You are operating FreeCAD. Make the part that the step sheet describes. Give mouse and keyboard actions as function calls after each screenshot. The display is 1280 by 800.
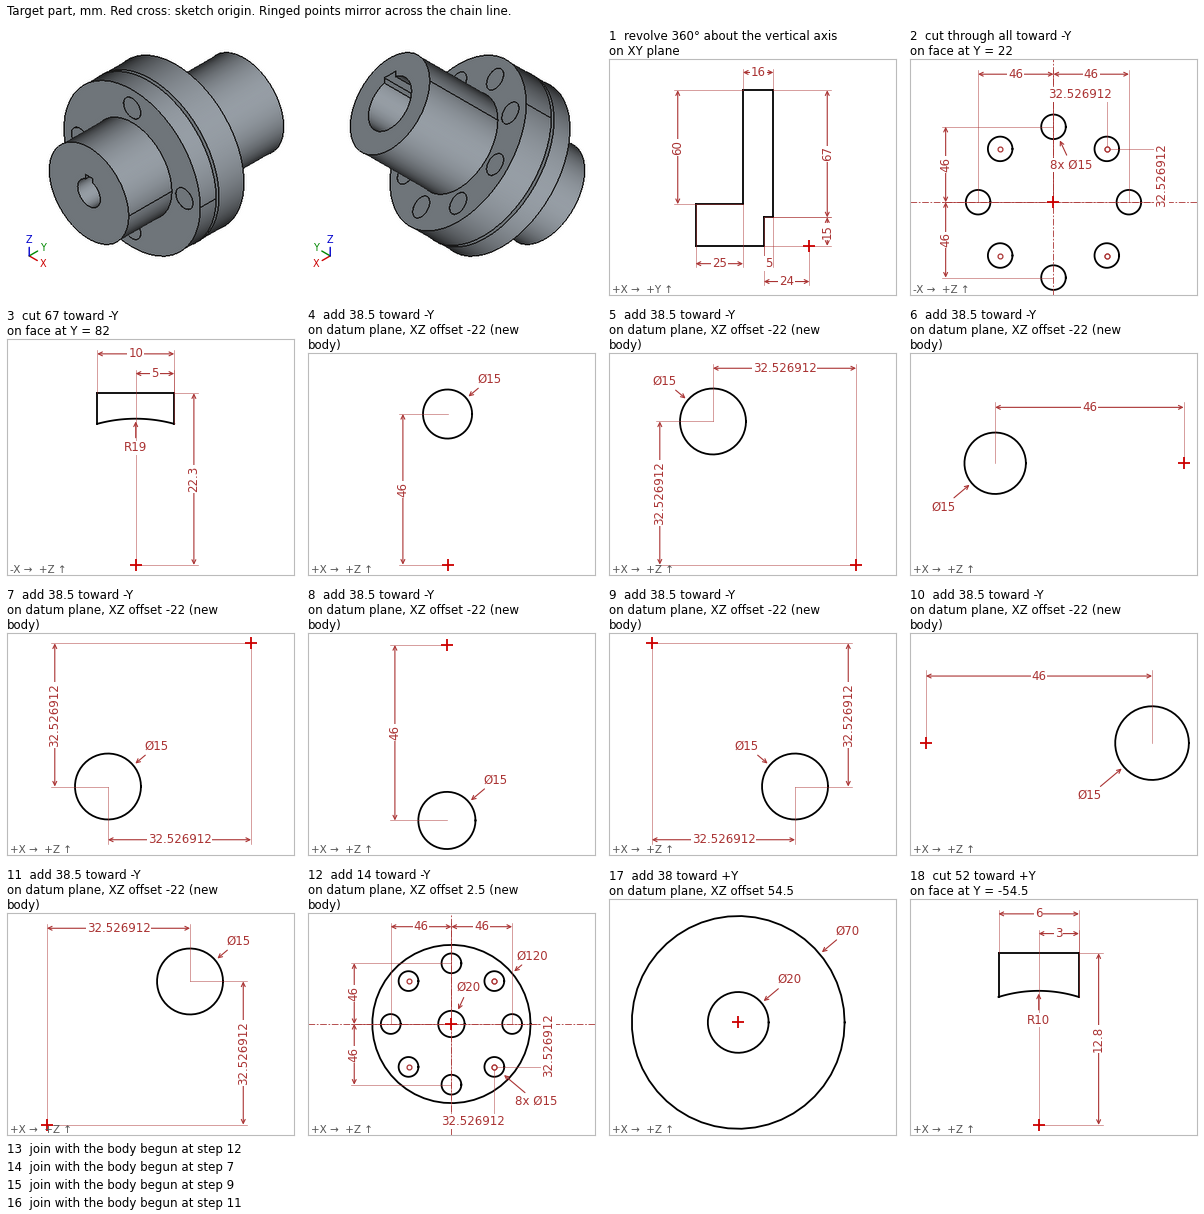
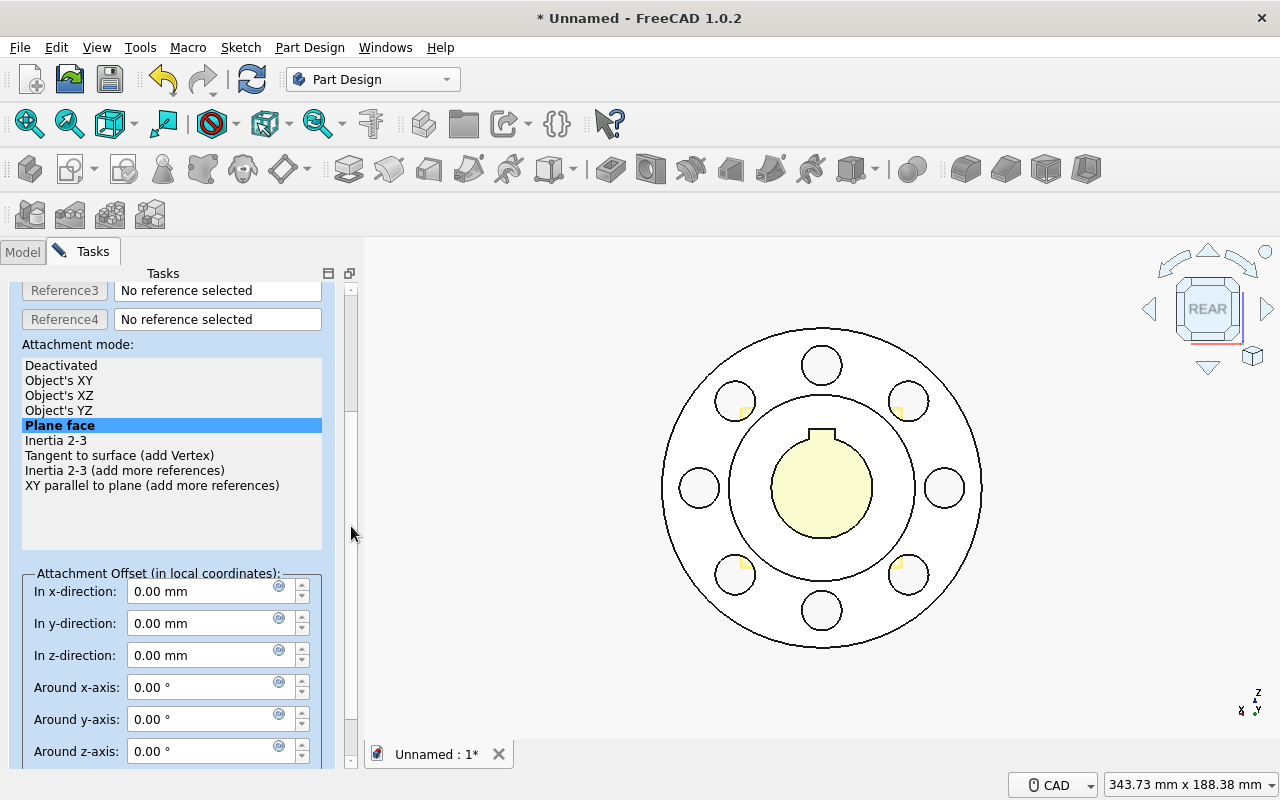
triple_click(210, 655)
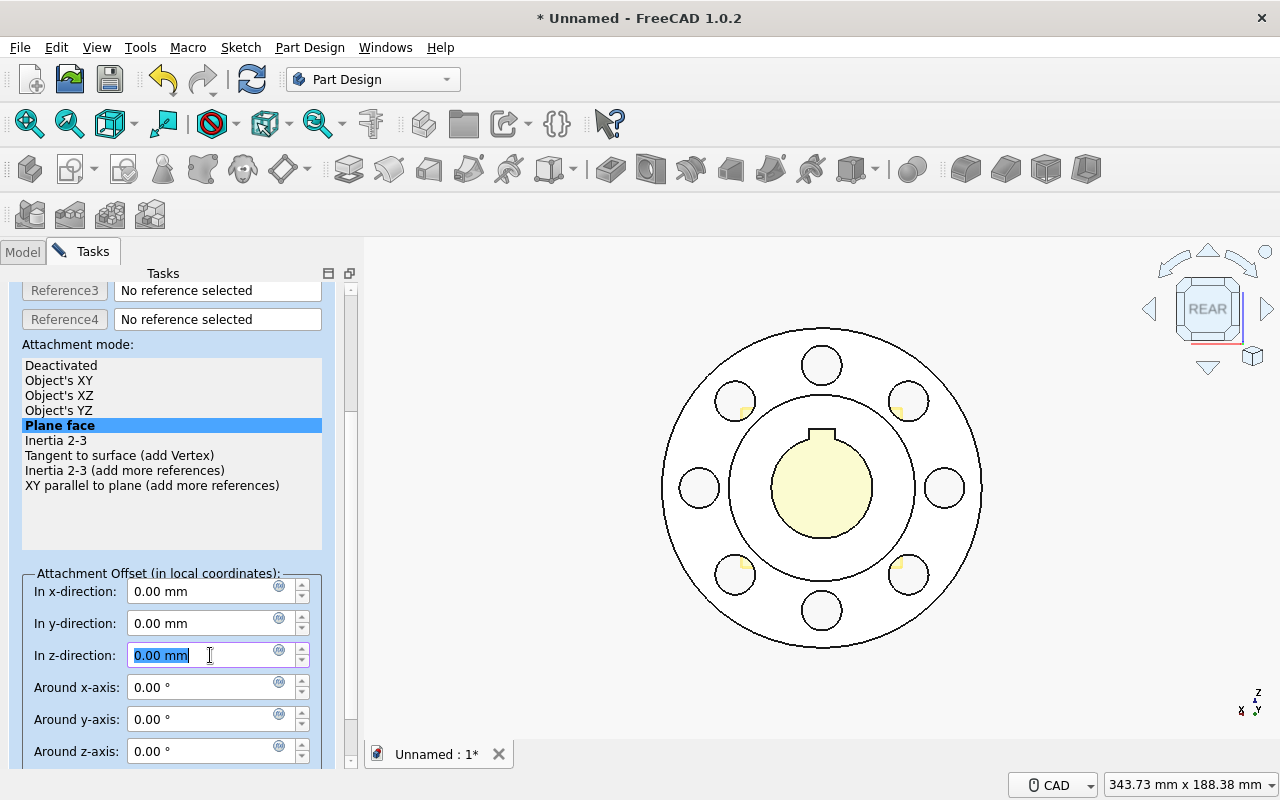
text(-22)
key(Tab)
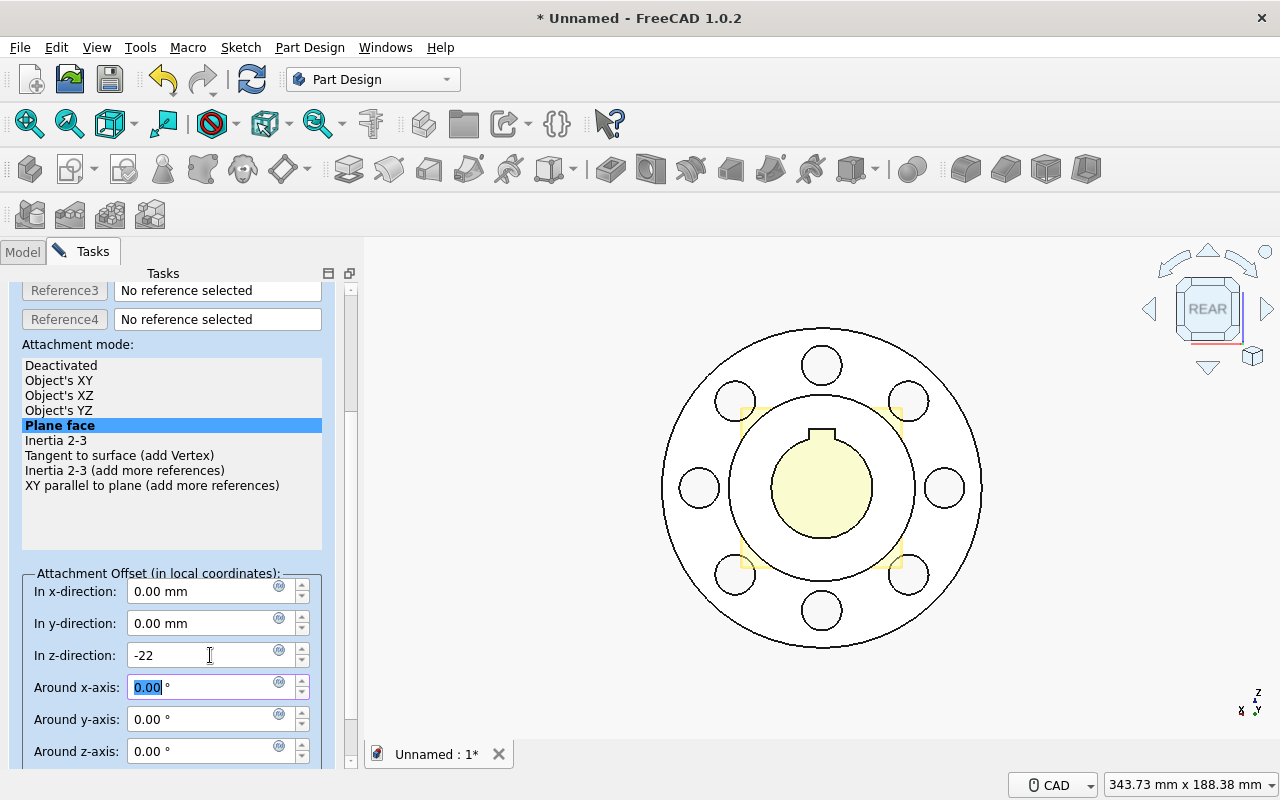
scroll(351, 526, up, 4)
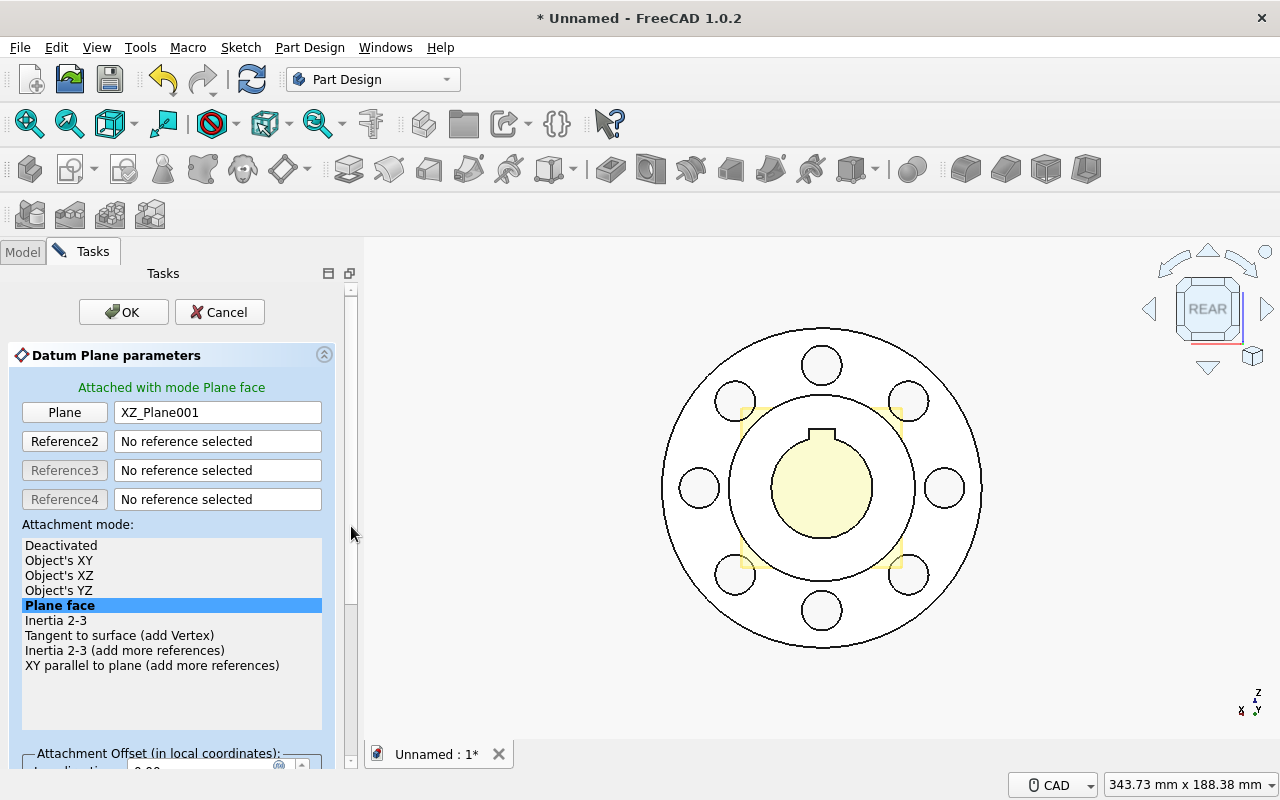
click(124, 312)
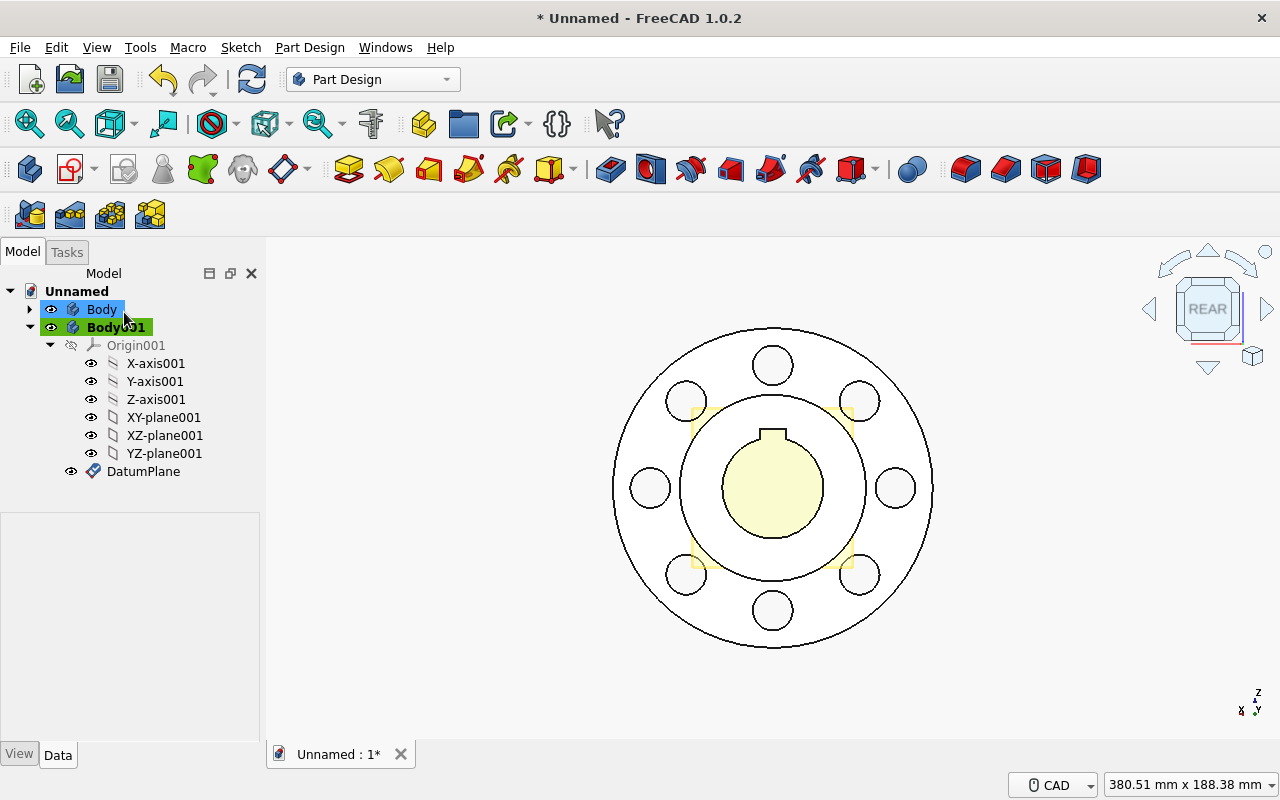
click(116, 471)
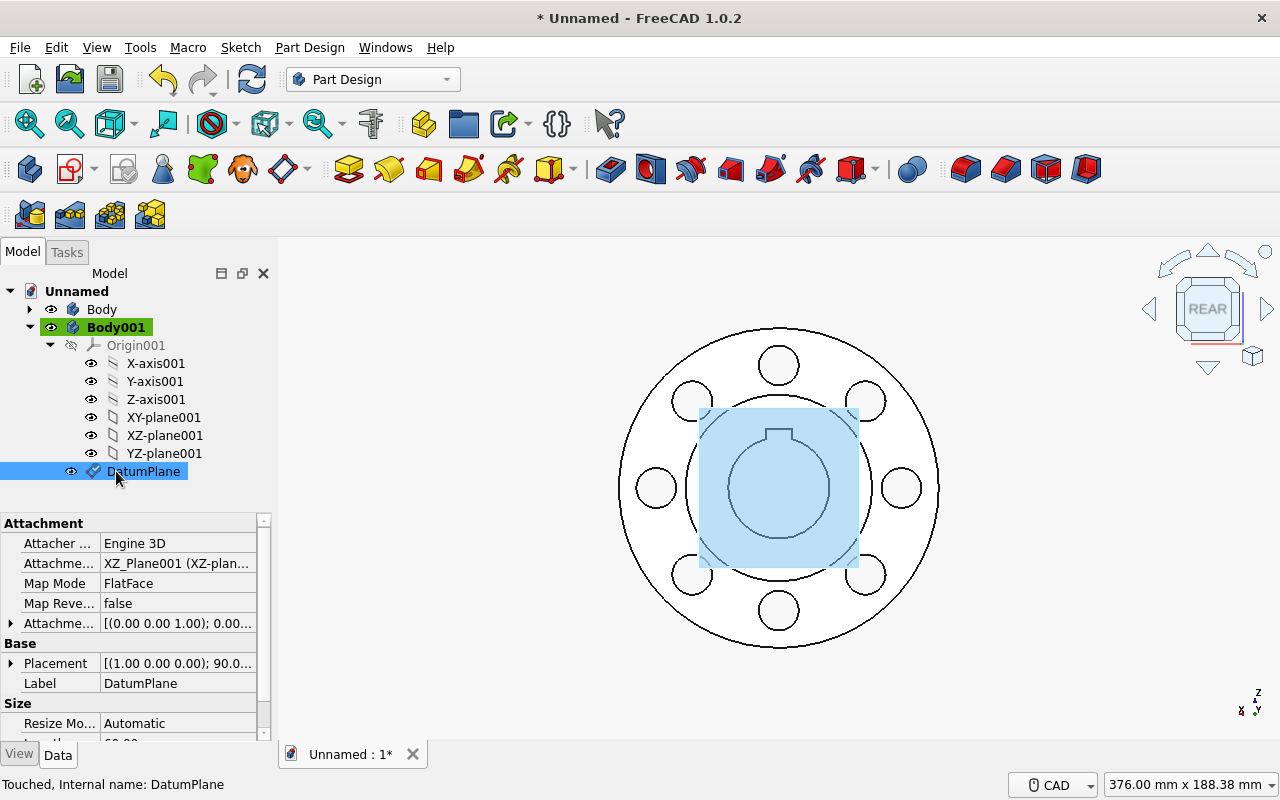
click(70, 170)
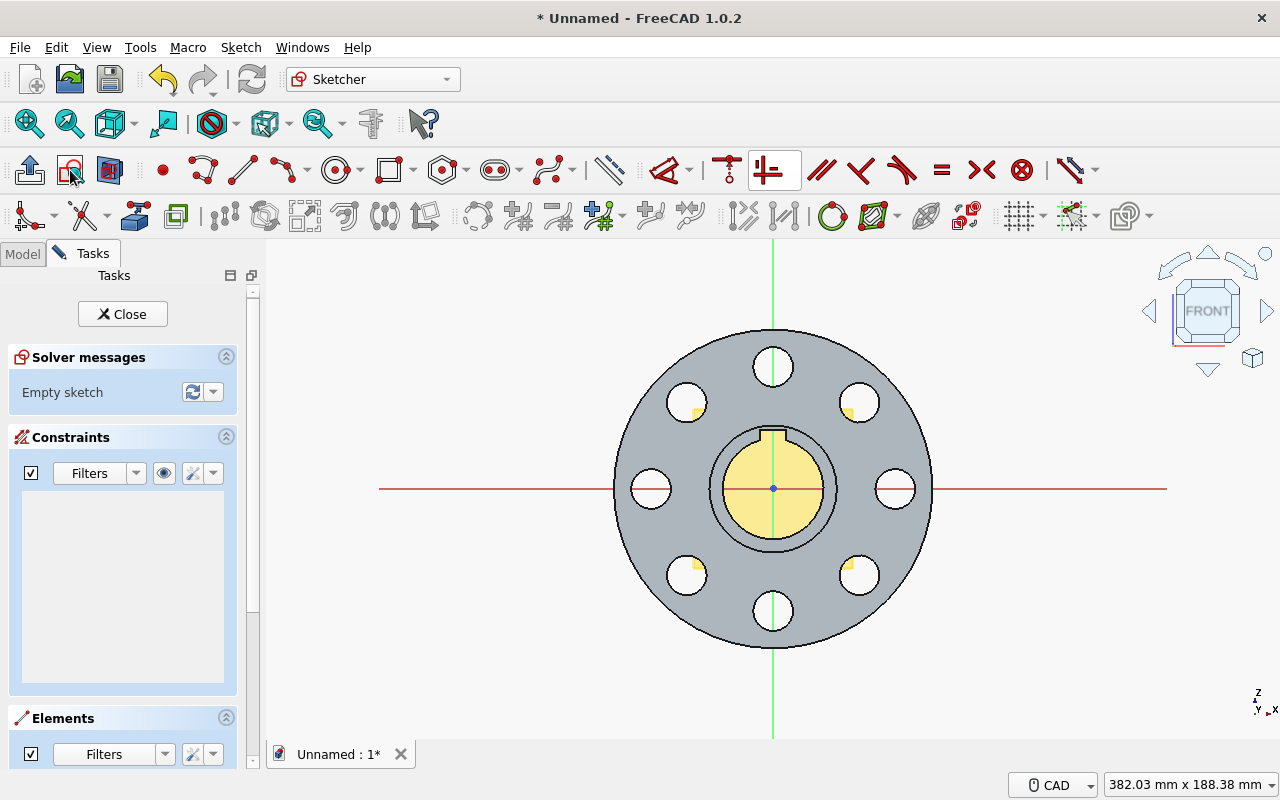
scroll(784, 348, up, 10)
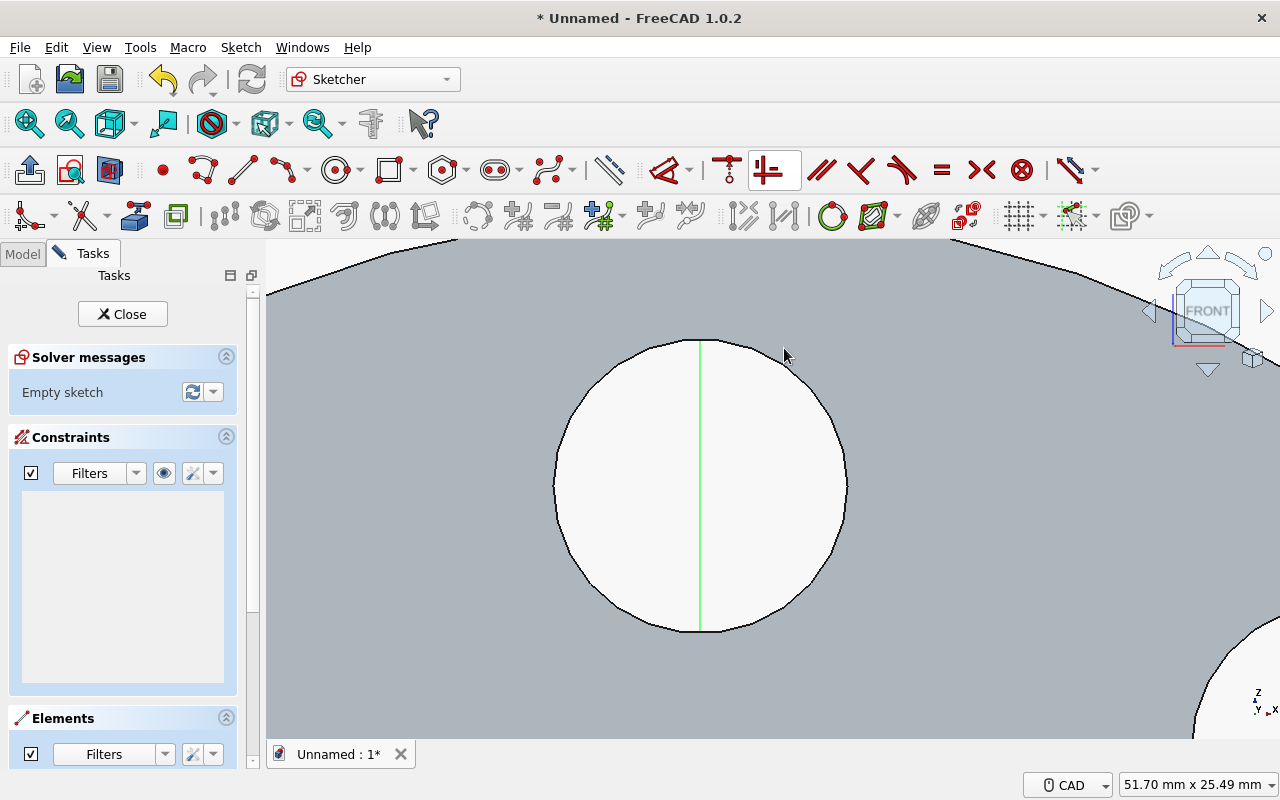
click(336, 170)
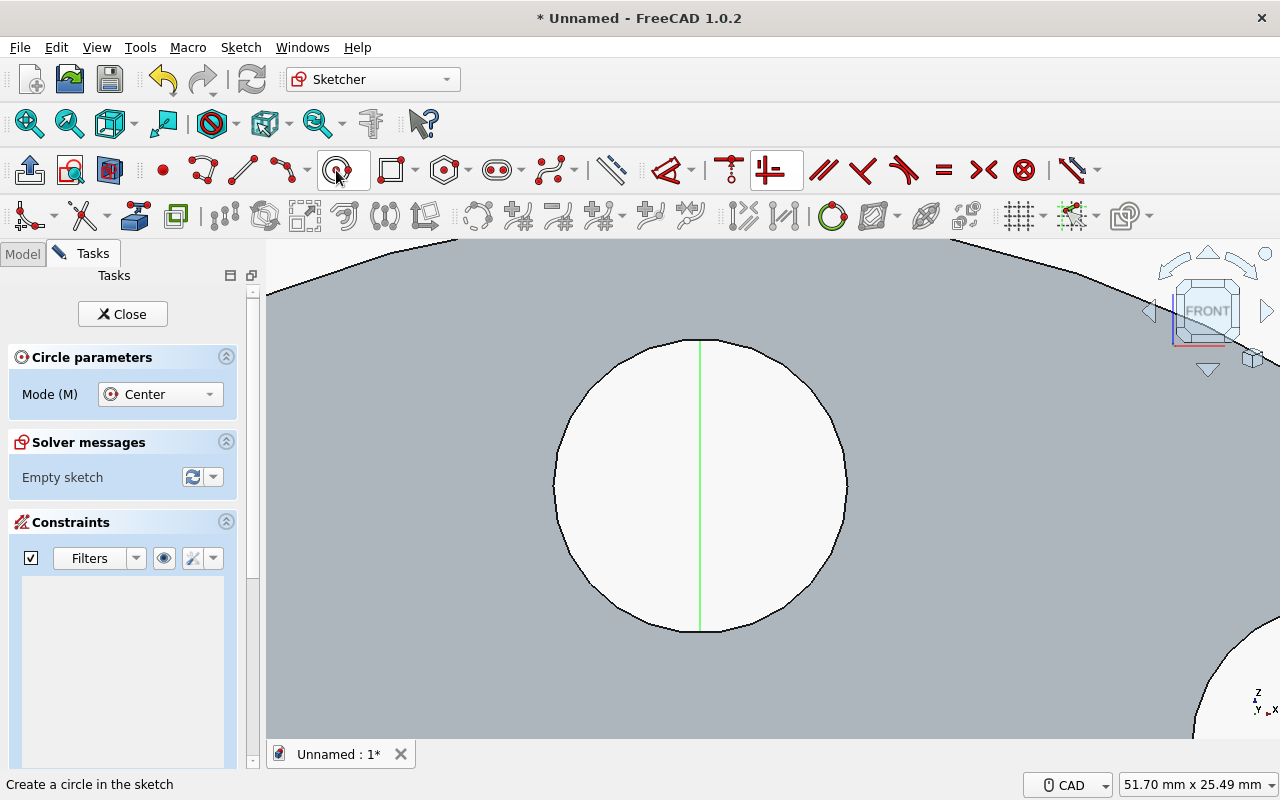
click(700, 486)
click(804, 382)
key(Escape)